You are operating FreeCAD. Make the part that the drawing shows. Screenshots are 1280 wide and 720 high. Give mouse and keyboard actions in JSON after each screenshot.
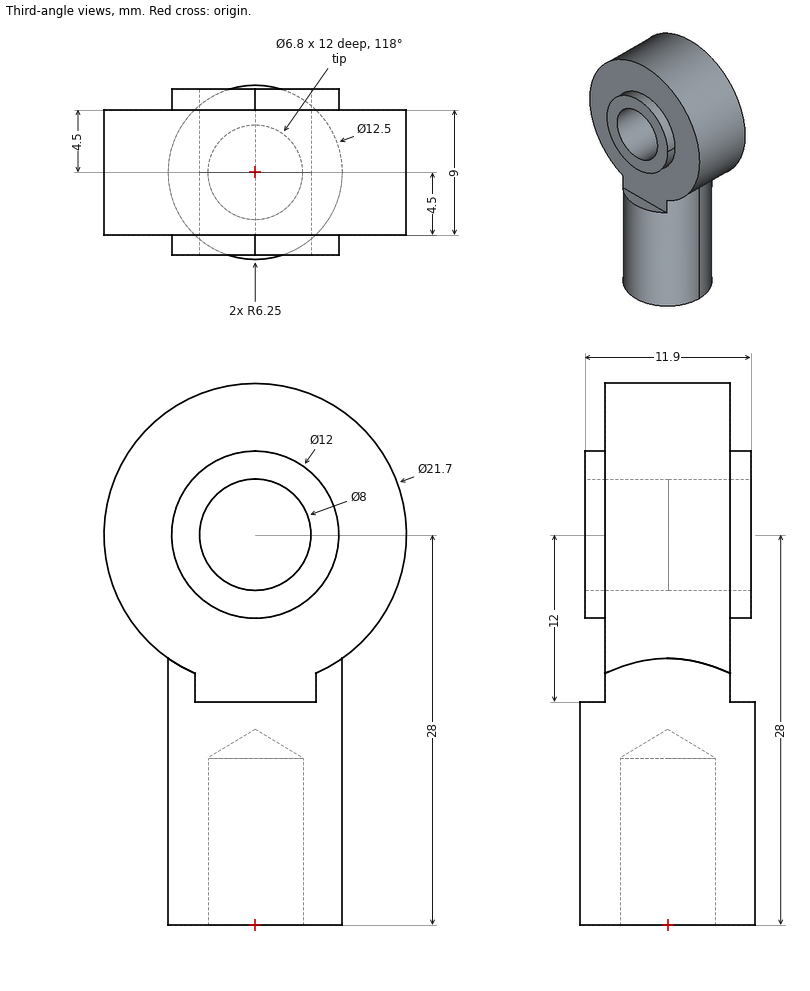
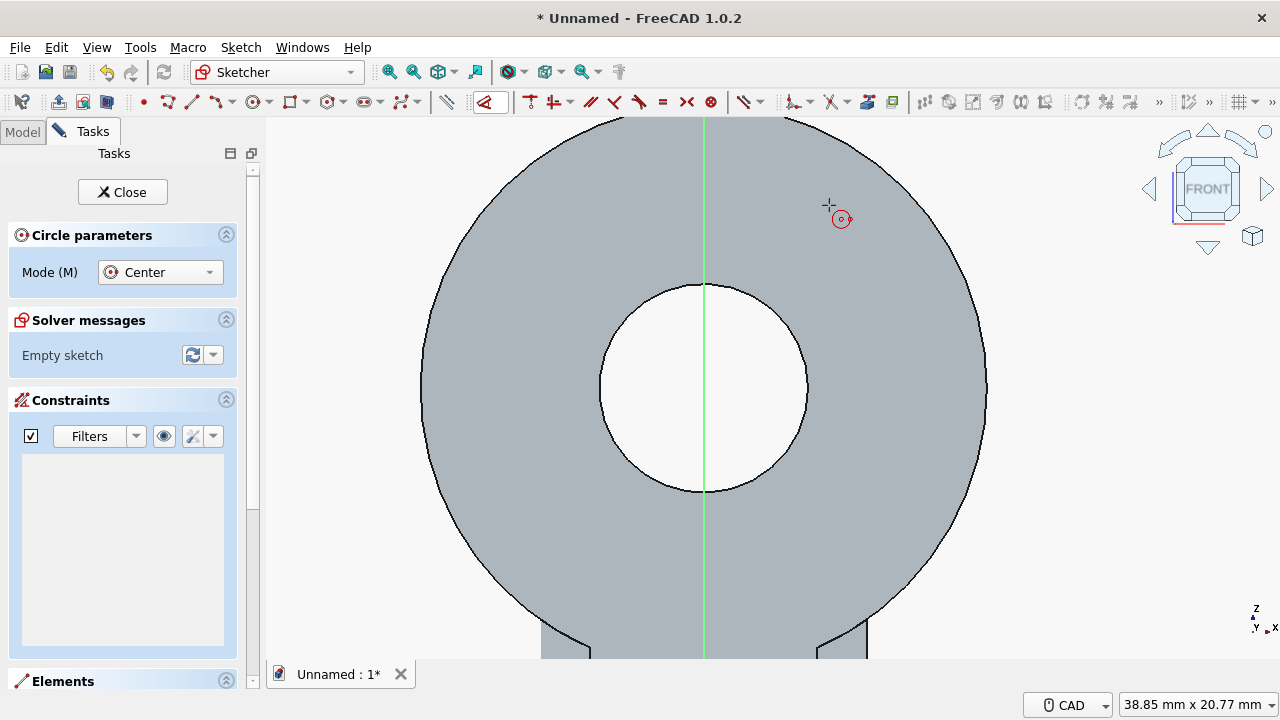
{"action": "left_click", "coordinate": [704, 388]}
{"action": "left_click", "coordinate": [814, 278]}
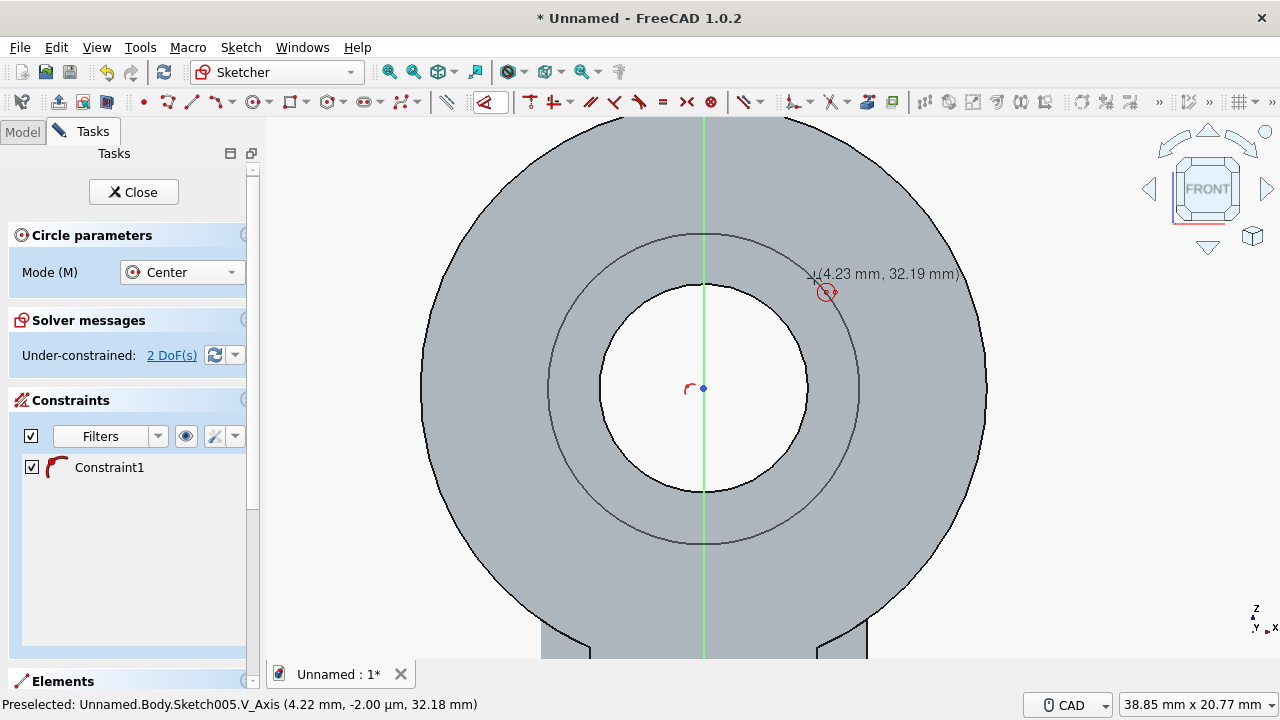
{"action": "left_click", "coordinate": [704, 389]}
{"action": "left_click", "coordinate": [777, 314]}
{"action": "key", "text": "Escape"}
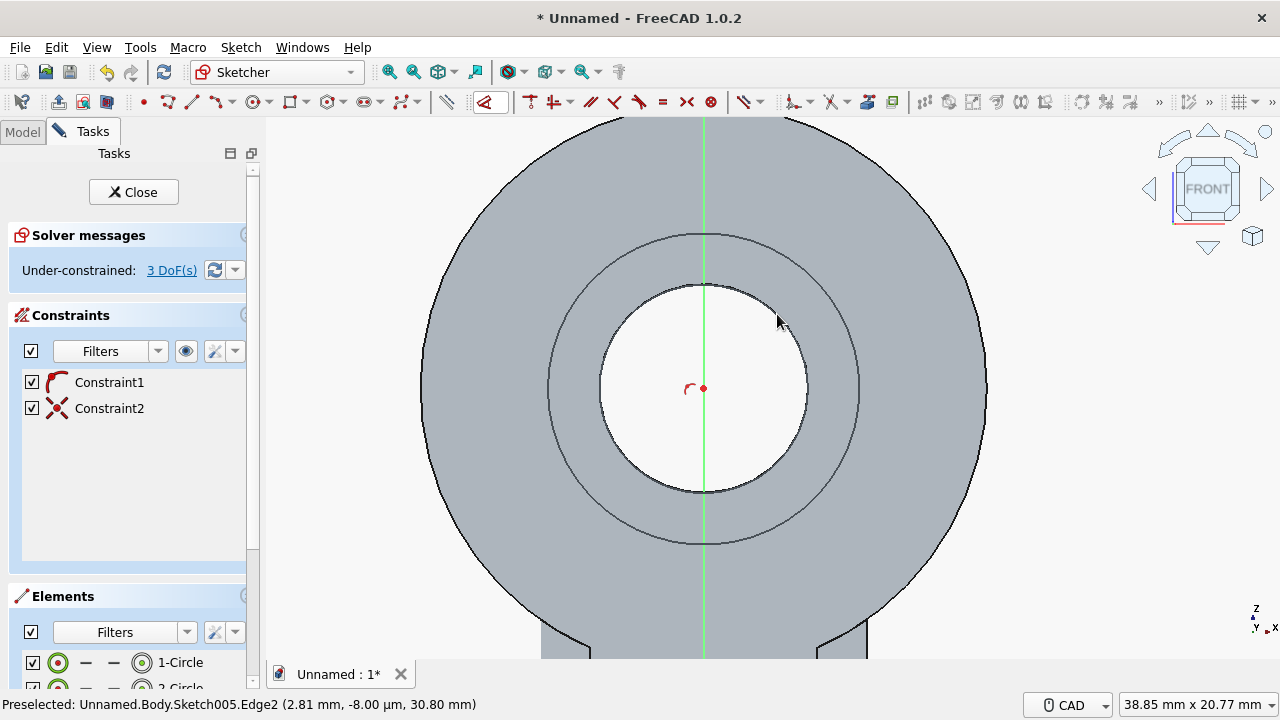
{"action": "left_click", "coordinate": [813, 278]}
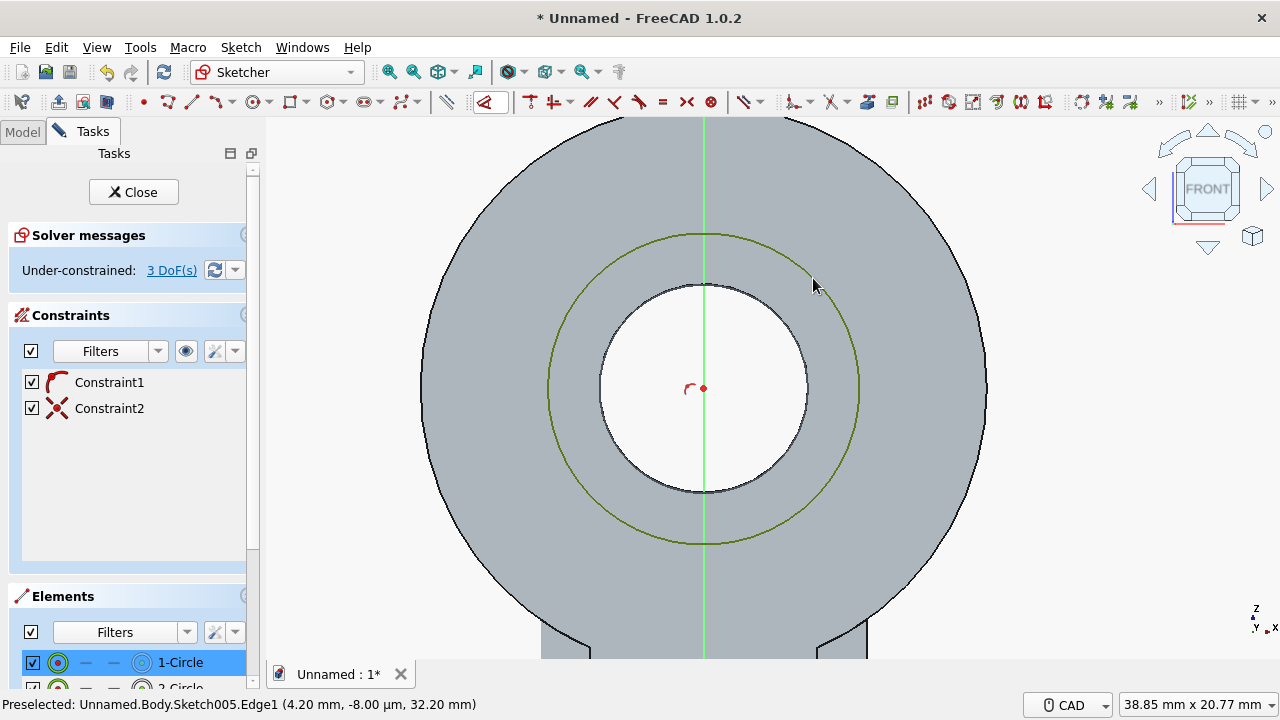
{"action": "key", "text": "k o"}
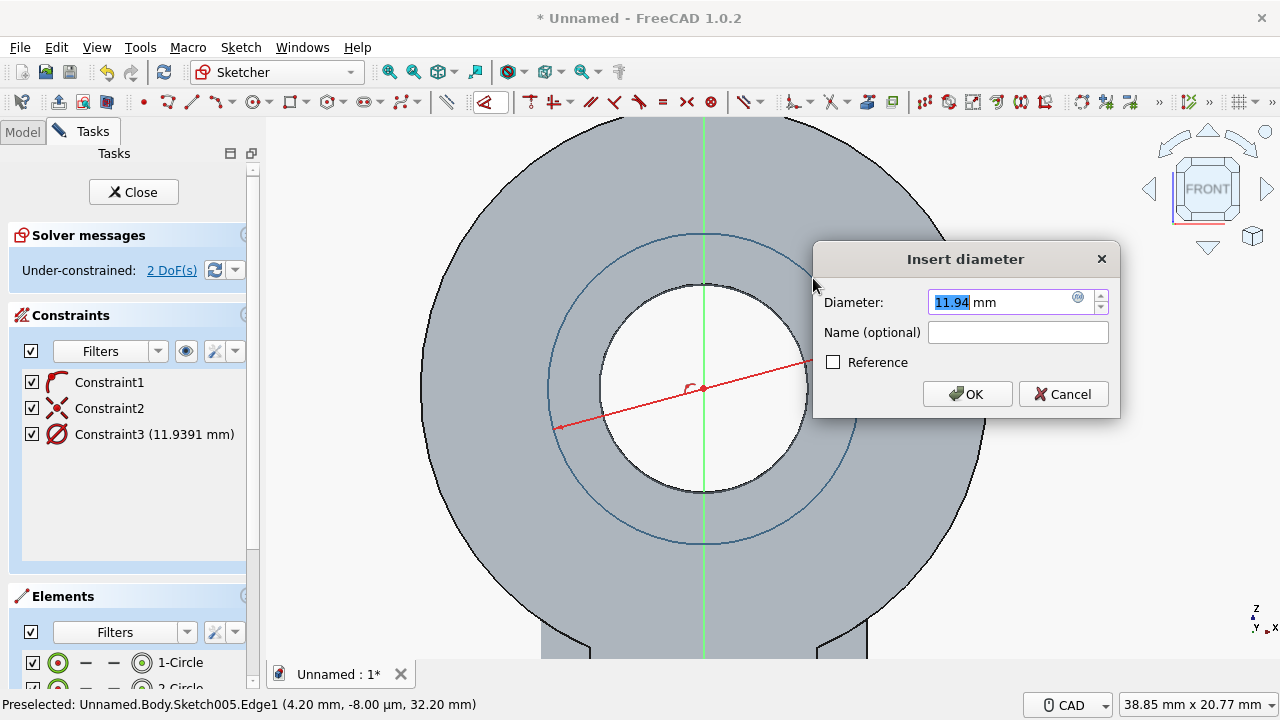
{"action": "type", "text": "12"}
{"action": "key", "text": "Return"}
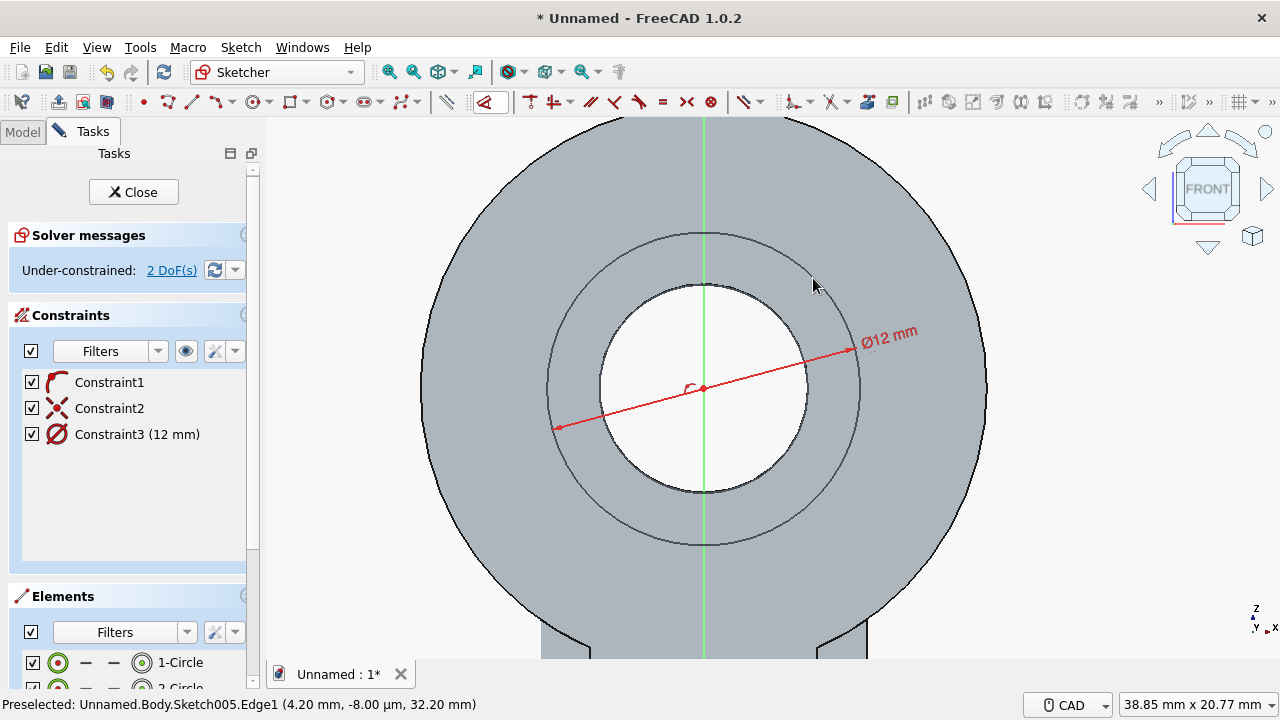
{"action": "left_click", "coordinate": [777, 315]}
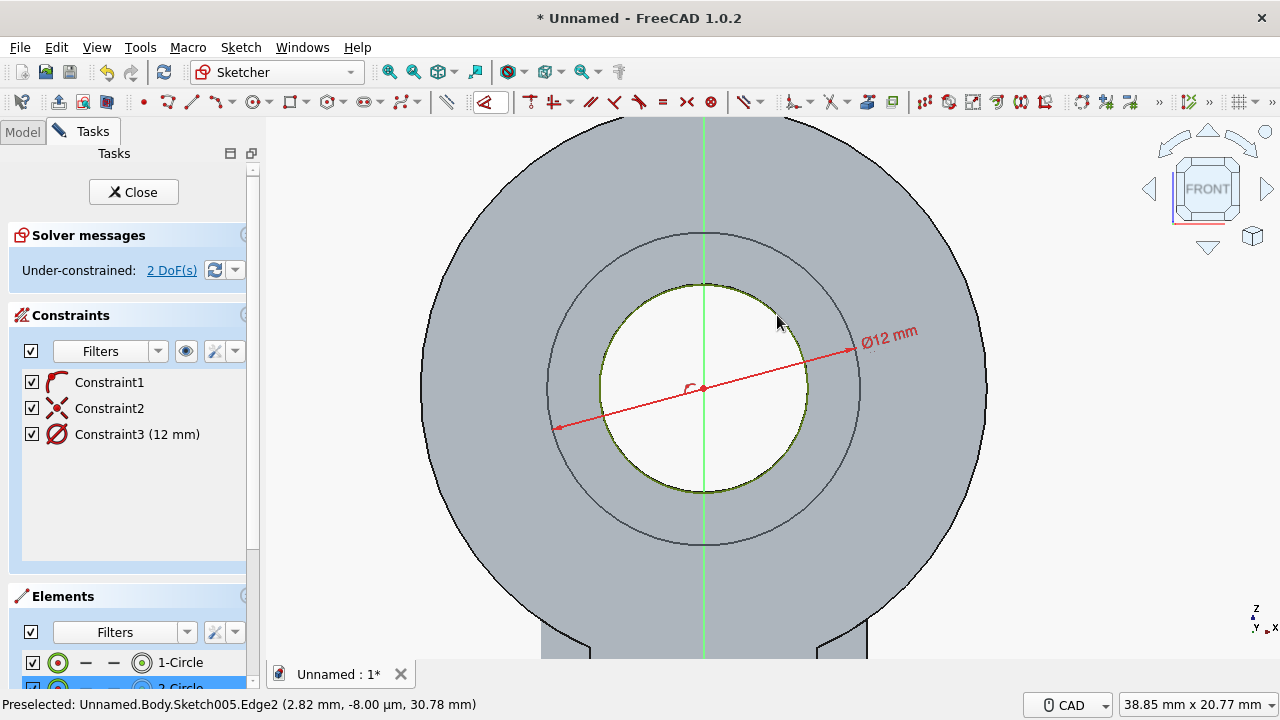
{"action": "key", "text": "k o"}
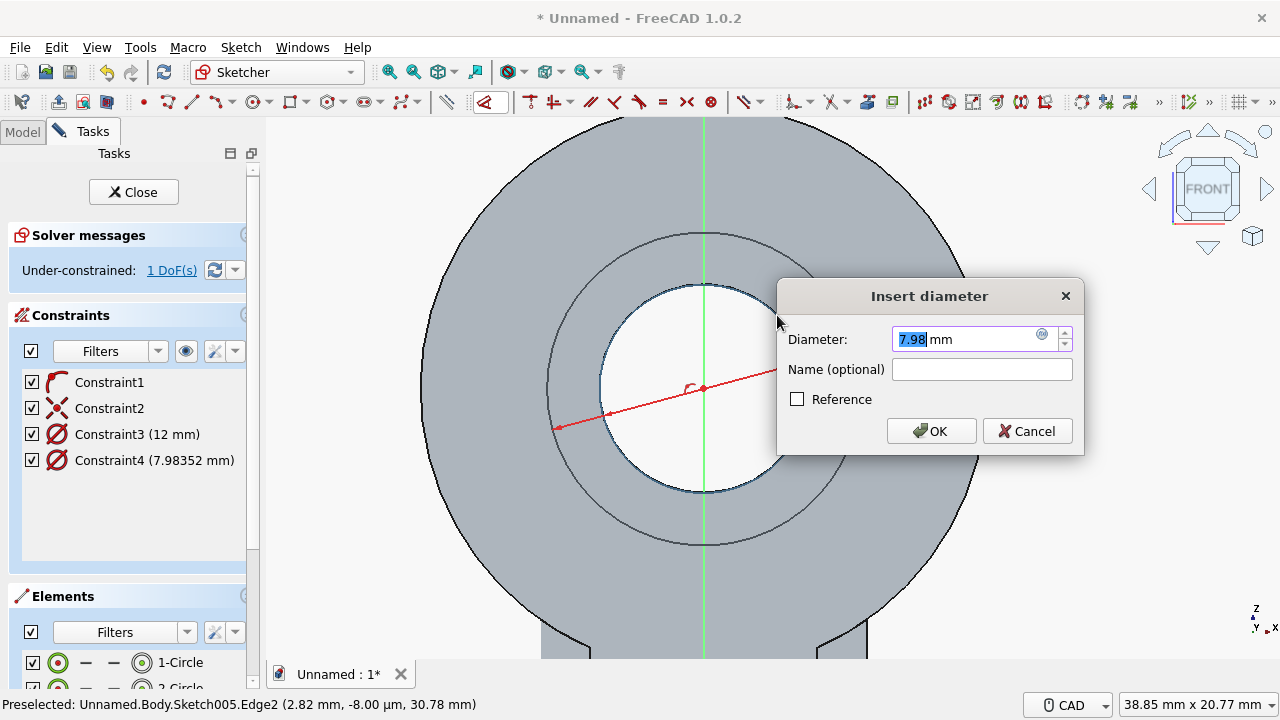
{"action": "type", "text": "8"}
{"action": "key", "text": "Return"}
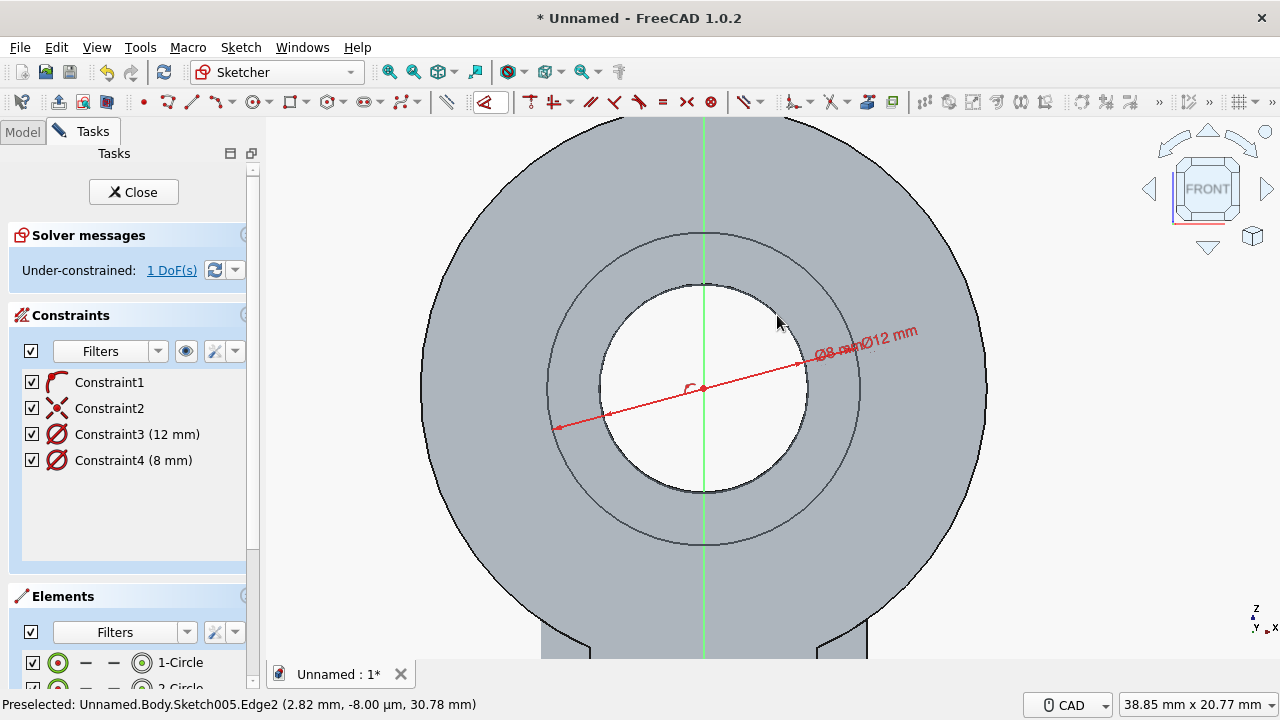
{"action": "left_click", "coordinate": [704, 389]}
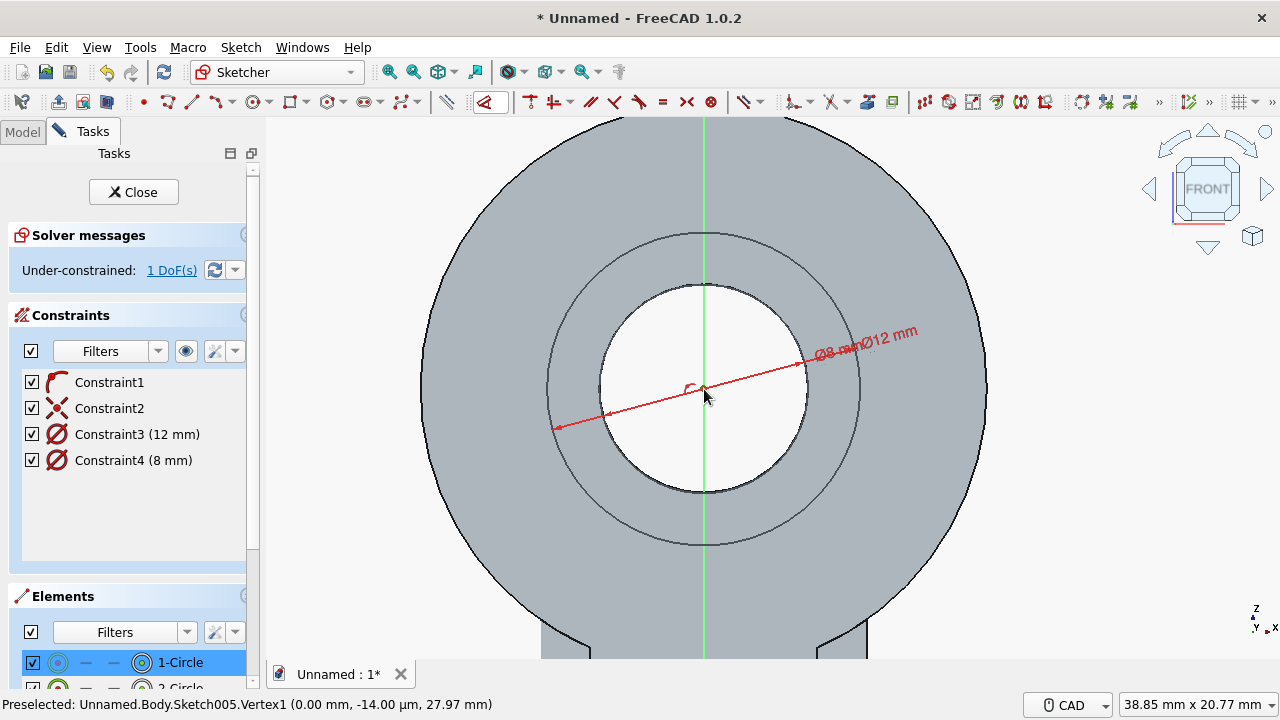
{"action": "key", "text": "i"}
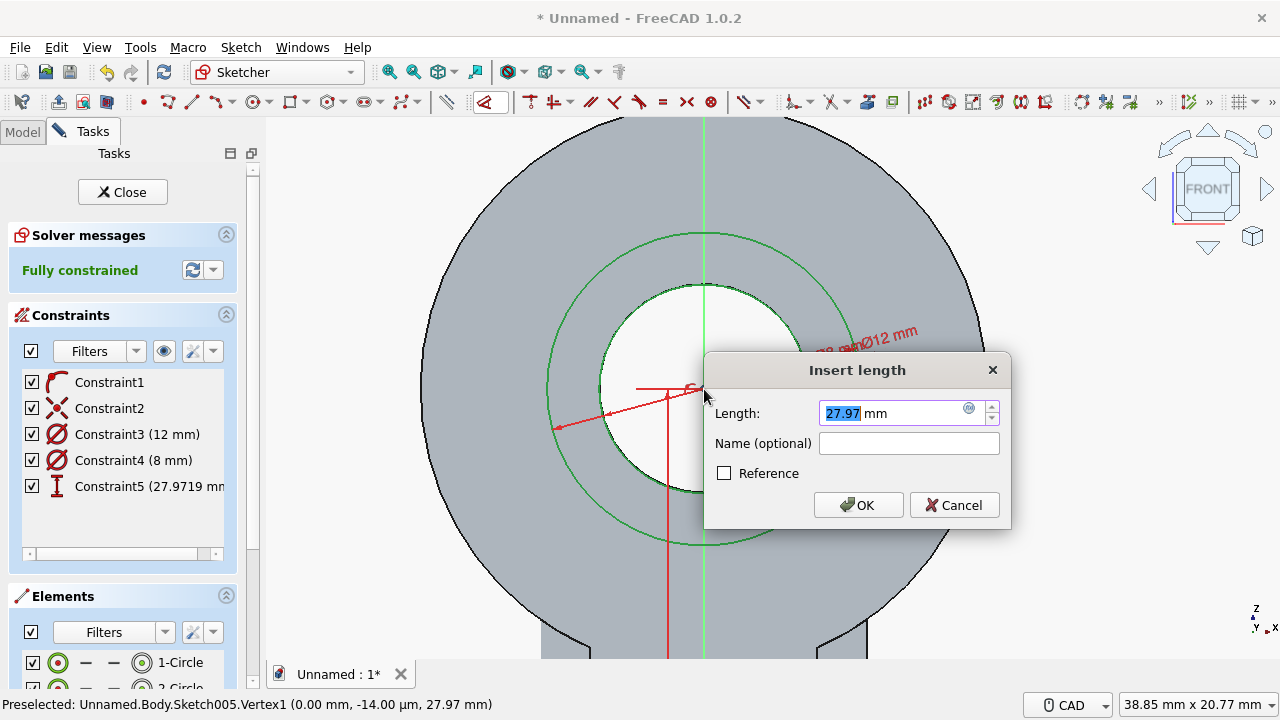
{"action": "type", "text": "28"}
{"action": "key", "text": "Return"}